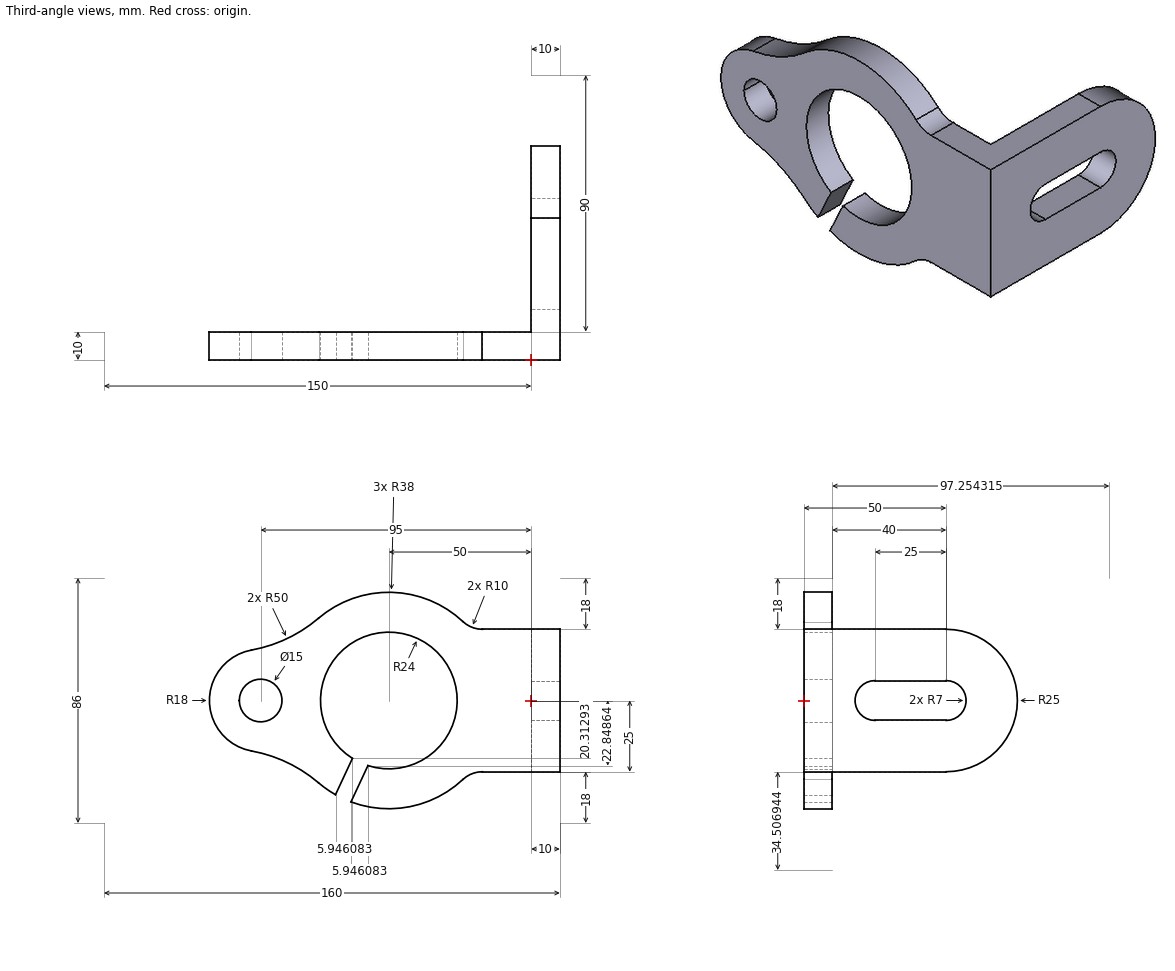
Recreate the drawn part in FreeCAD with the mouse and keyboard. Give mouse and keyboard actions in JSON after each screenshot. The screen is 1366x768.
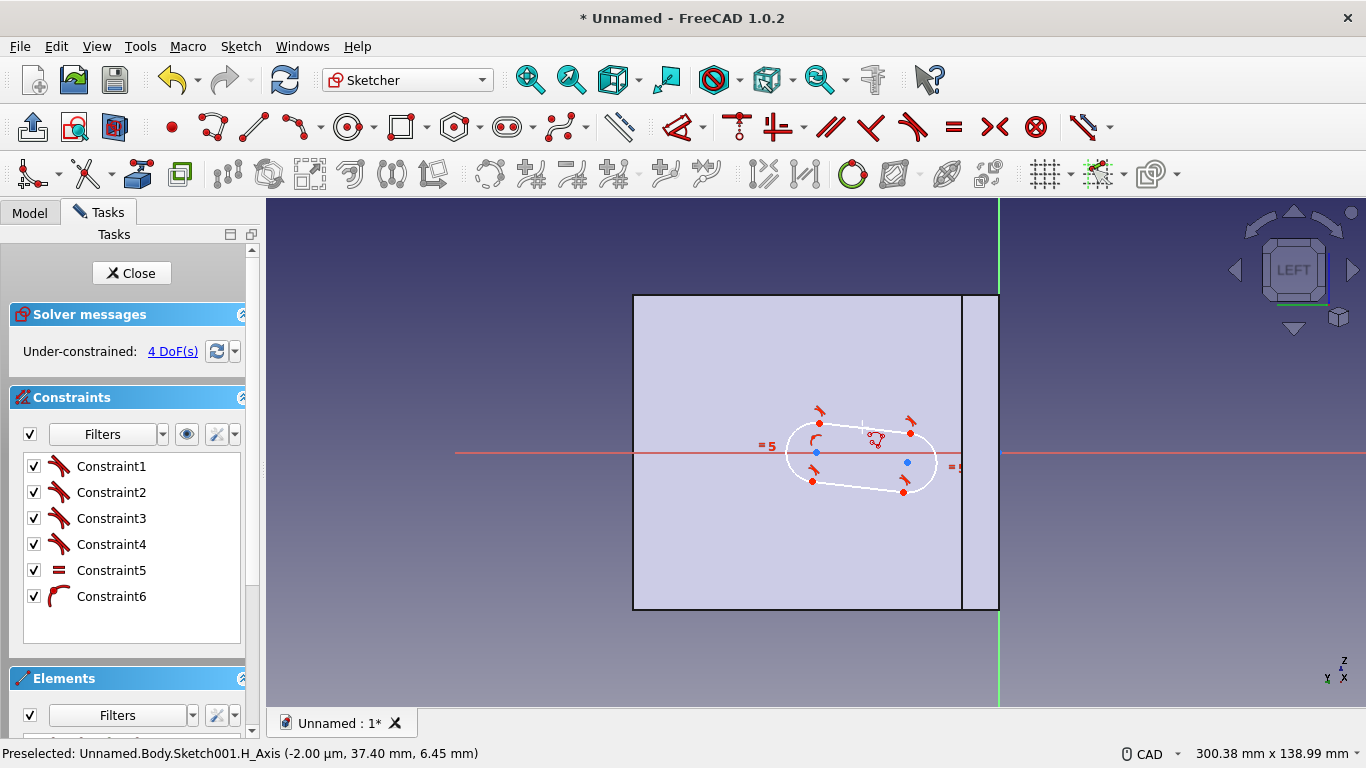
{"action": "left_click", "coordinate": [816, 361]}
{"action": "left_click", "coordinate": [962, 361]}
{"action": "left_click", "coordinate": [962, 295]}
{"action": "left_click", "coordinate": [606, 295]}
{"action": "left_click", "coordinate": [606, 670]}
{"action": "left_click", "coordinate": [962, 670]}
{"action": "left_click", "coordinate": [962, 544]}
{"action": "left_click", "coordinate": [816, 544]}
{"action": "right_click", "coordinate": [816, 544]}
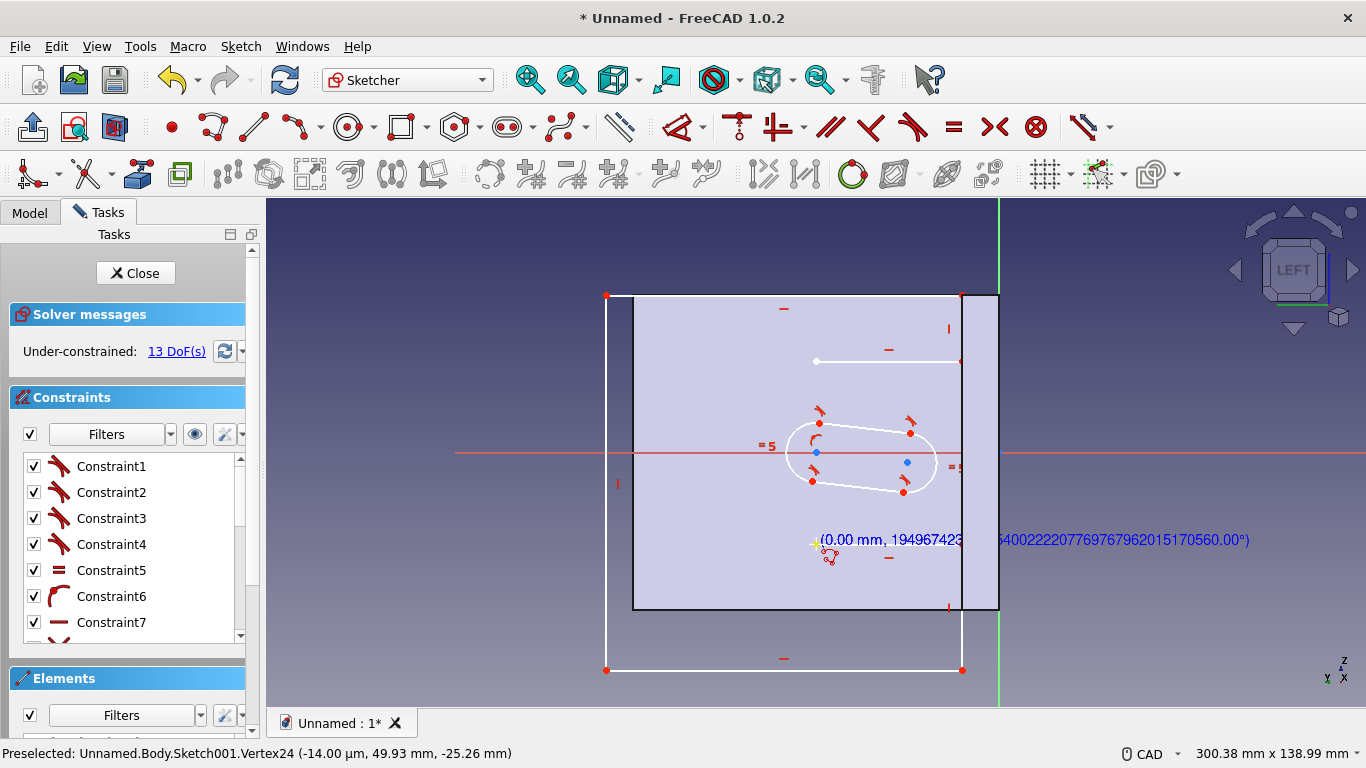
{"action": "key", "text": "g 3 a"}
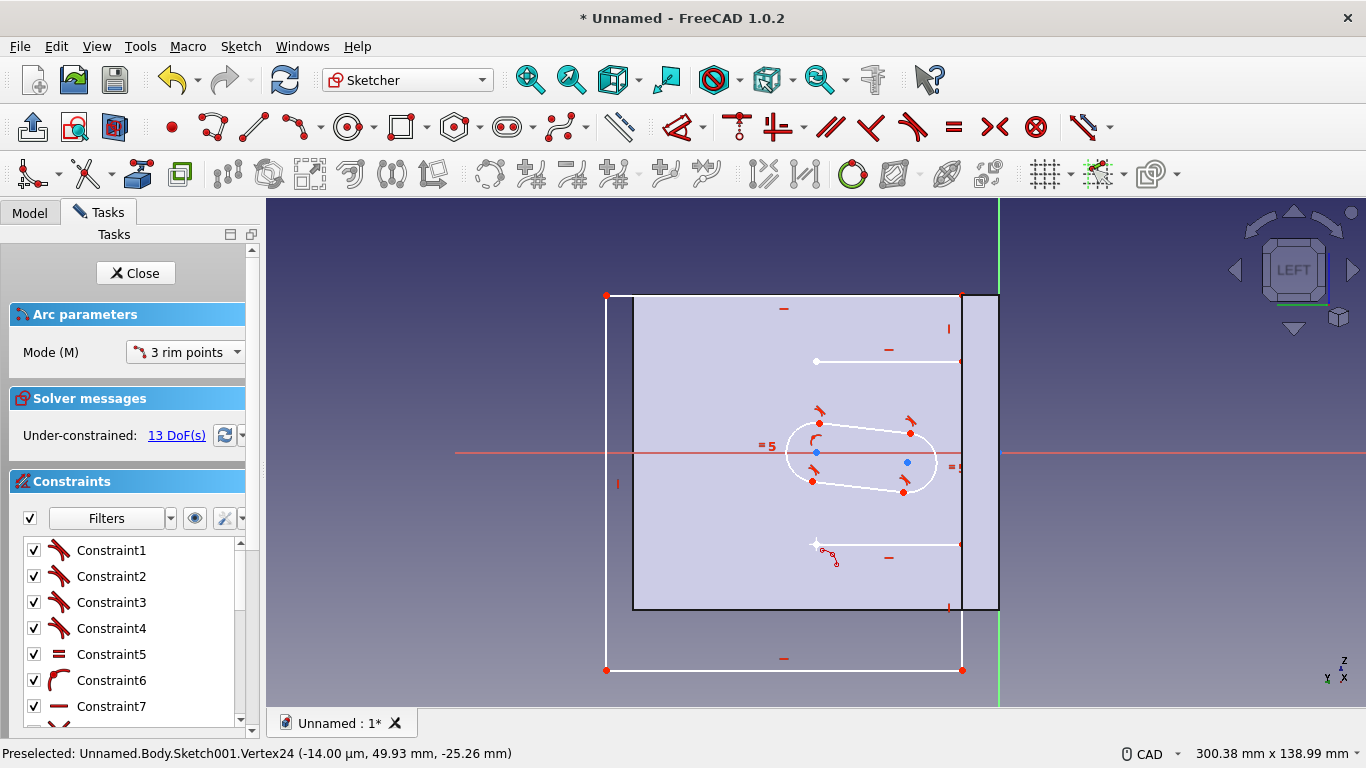
{"action": "left_click", "coordinate": [816, 545]}
{"action": "left_click", "coordinate": [816, 362]}
{"action": "left_click", "coordinate": [729, 424]}
{"action": "key", "text": "Escape"}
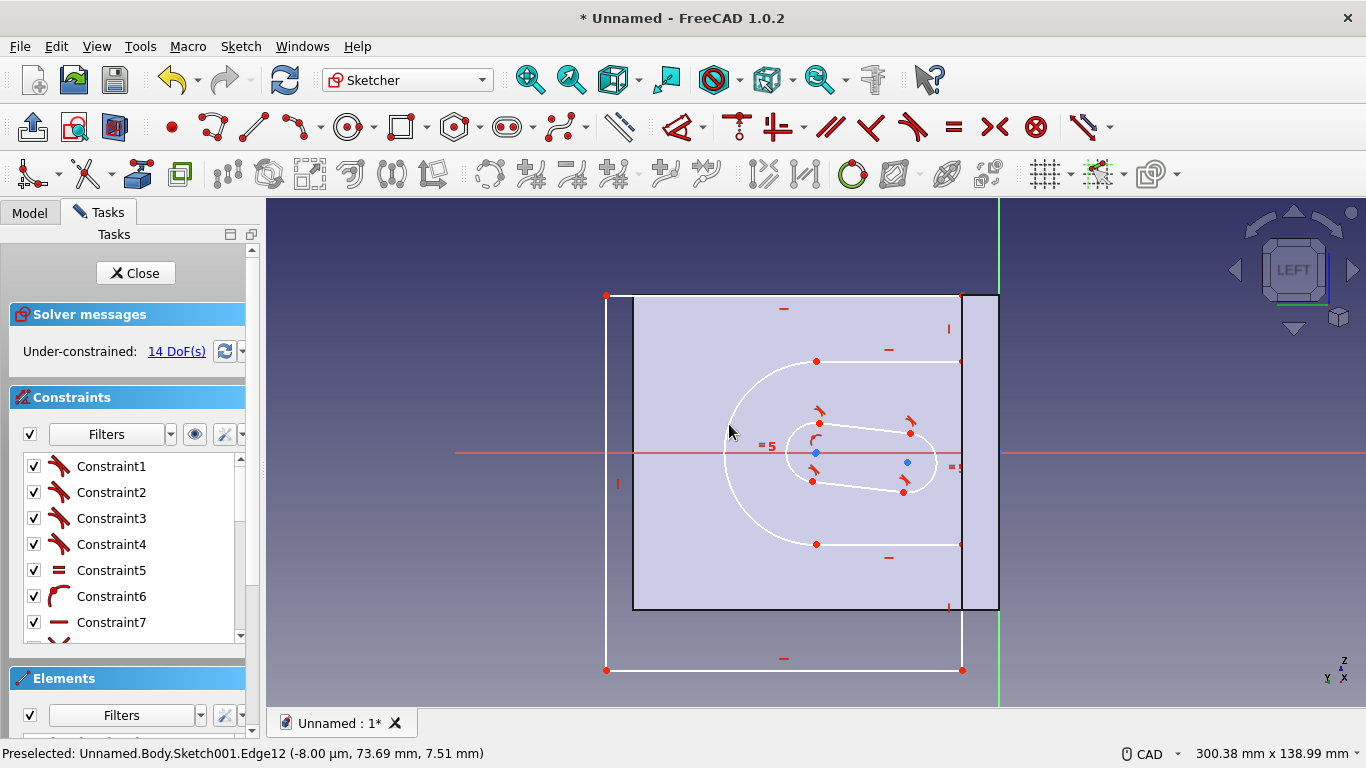
{"action": "left_click", "coordinate": [860, 362]}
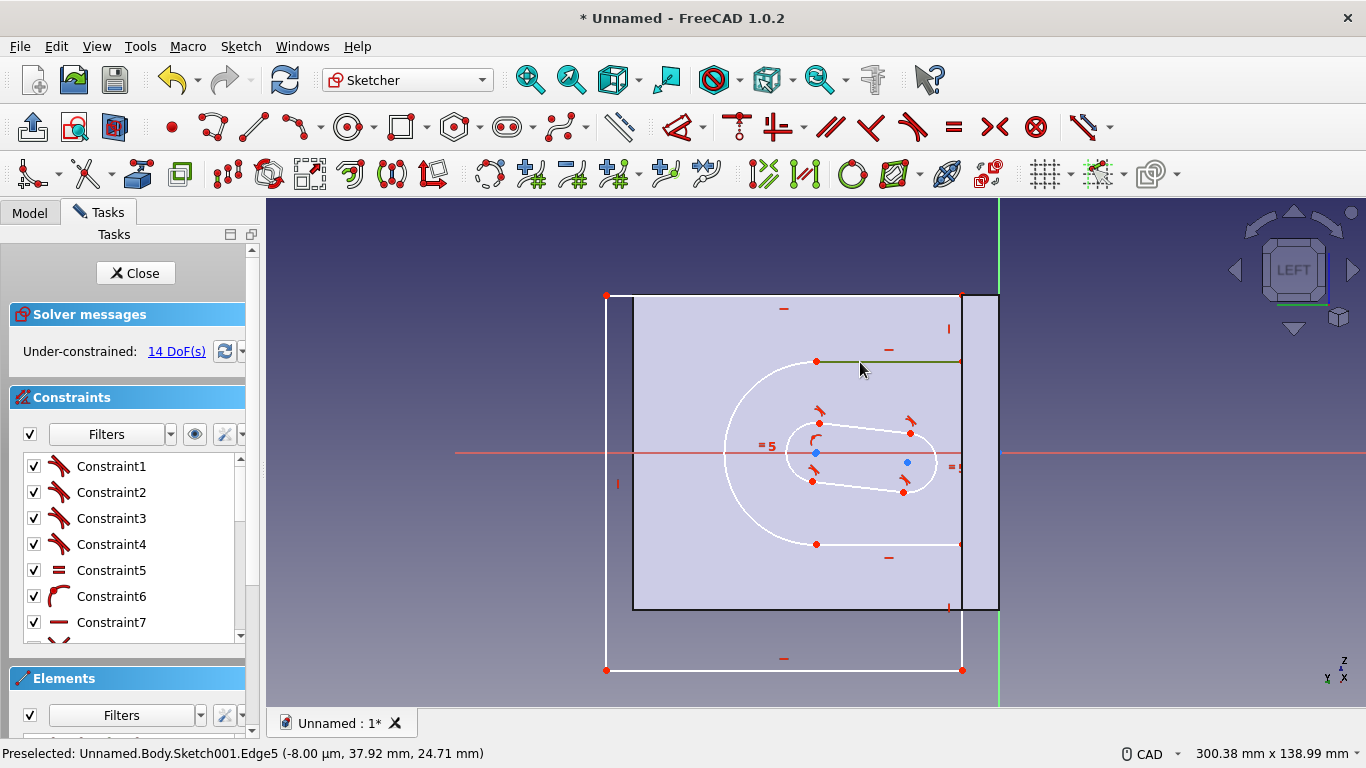
{"action": "left_click", "coordinate": [742, 400]}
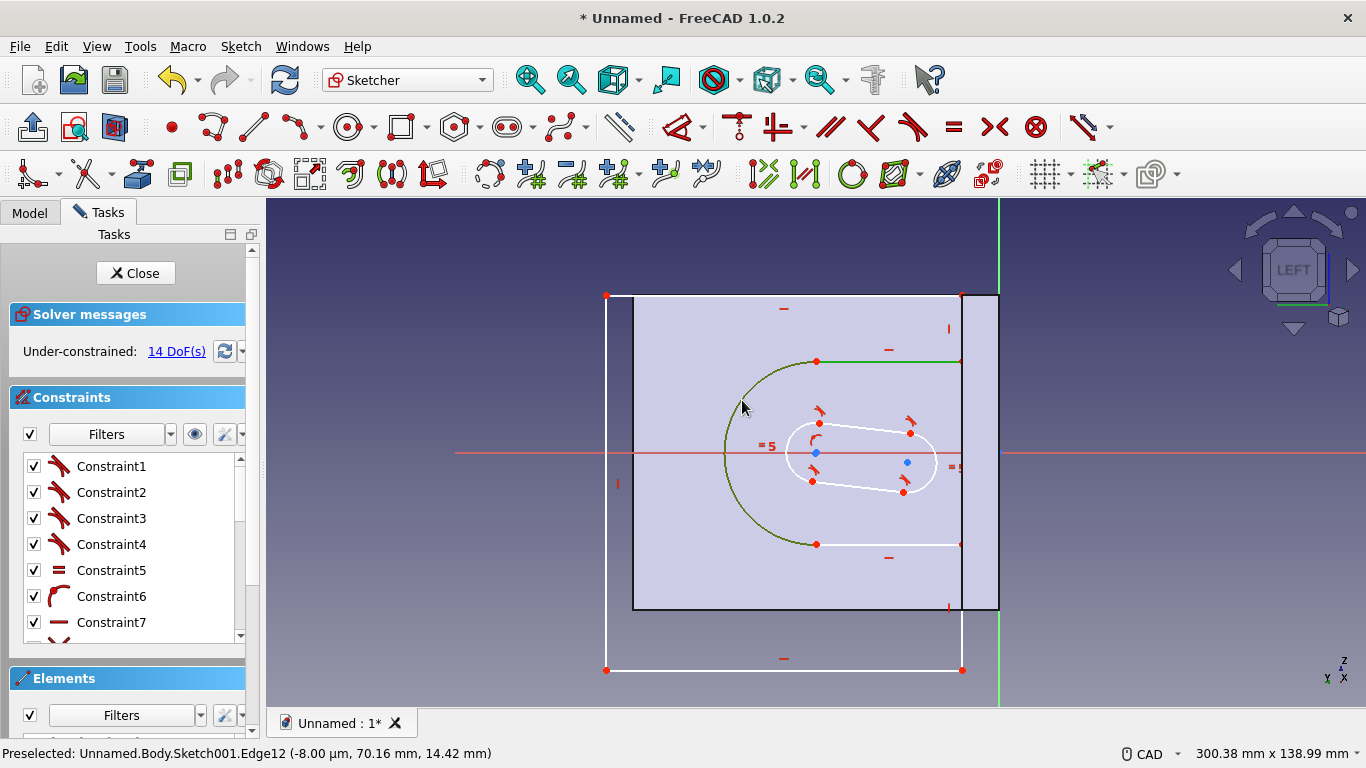
{"action": "key", "text": "t"}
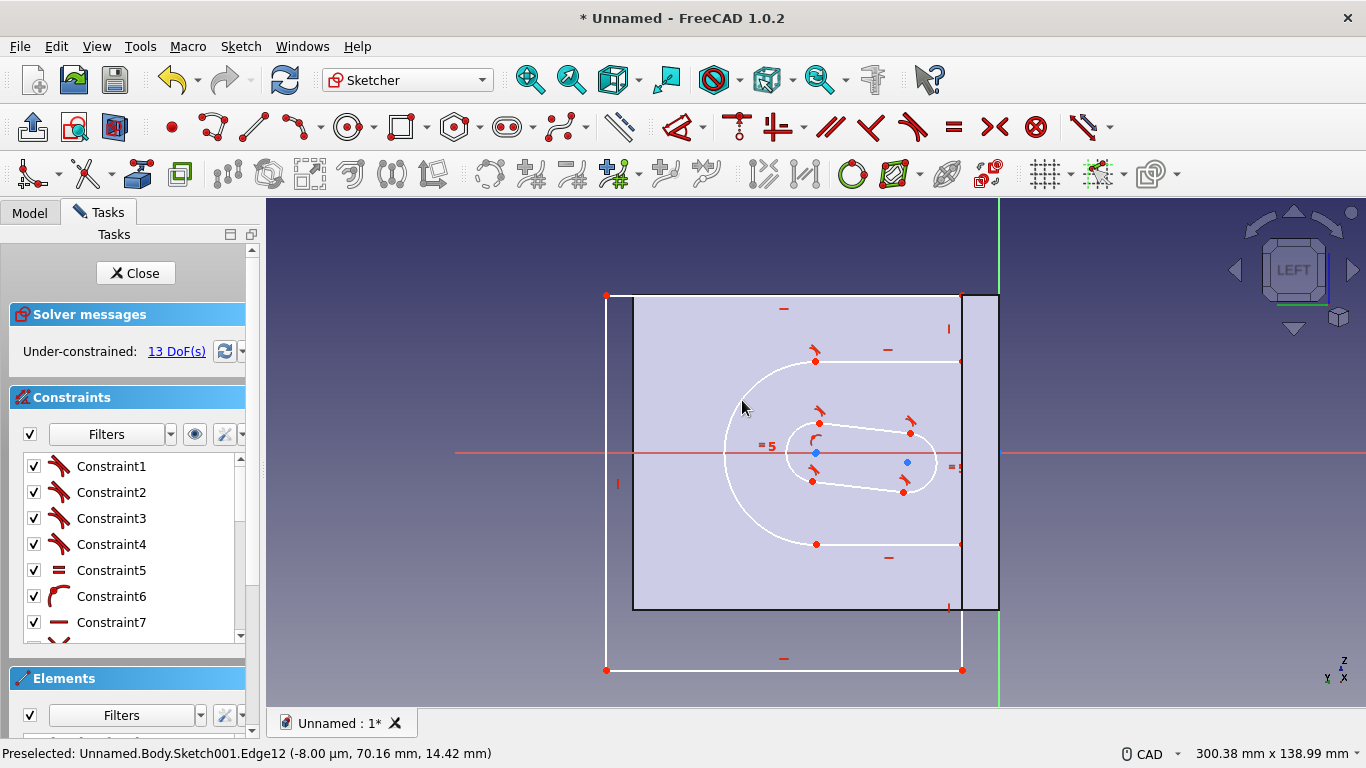
{"action": "left_click", "coordinate": [918, 545]}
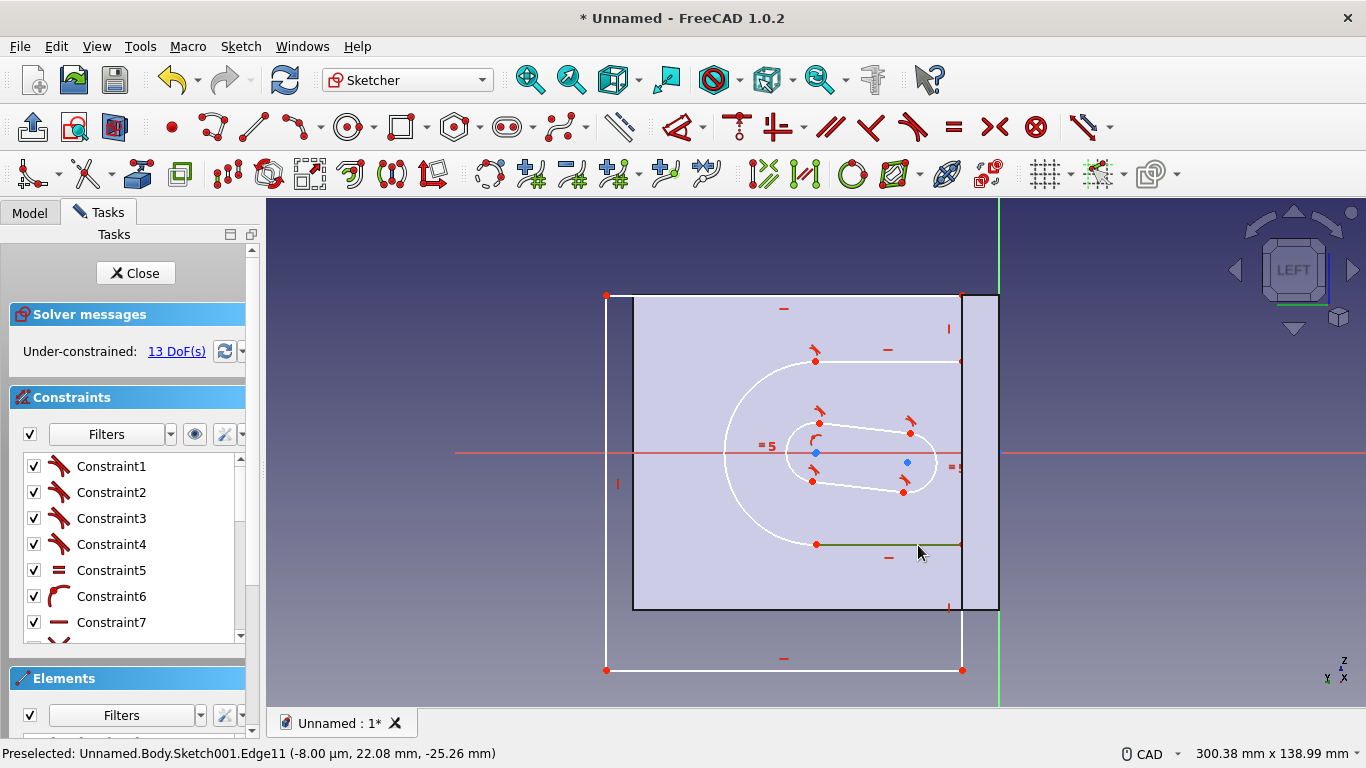
{"action": "left_click", "coordinate": [742, 400]}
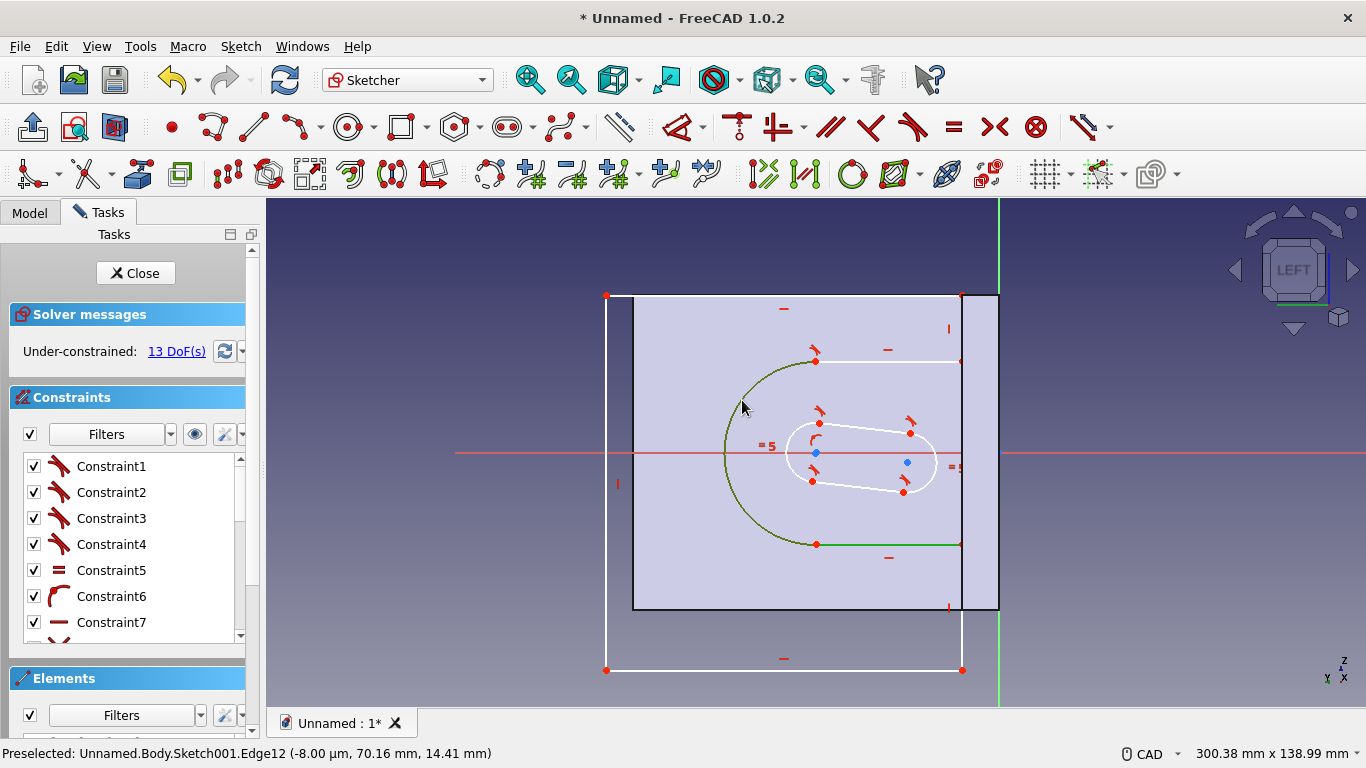
{"action": "left_click", "coordinate": [913, 128]}